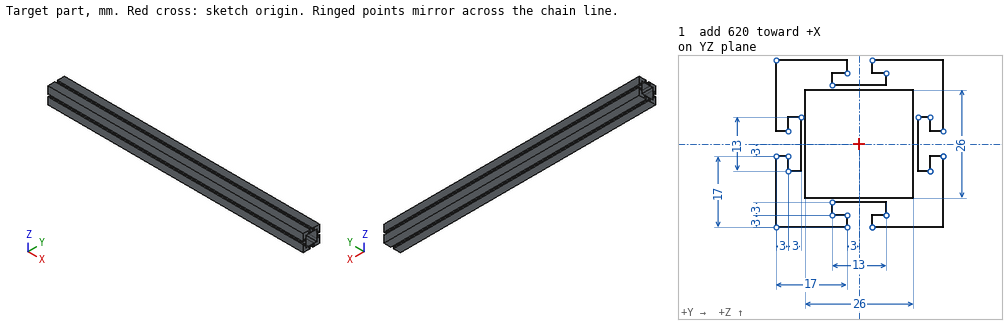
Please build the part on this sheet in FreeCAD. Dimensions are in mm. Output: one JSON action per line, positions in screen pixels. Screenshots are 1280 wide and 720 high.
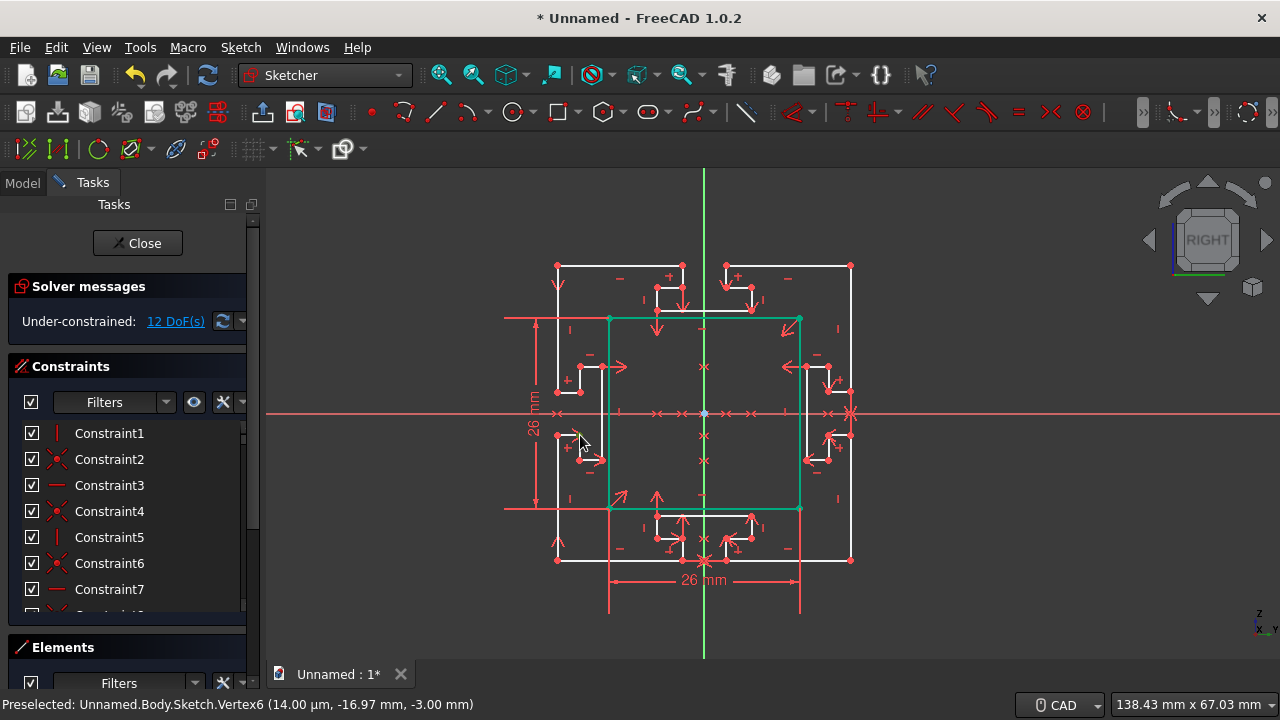
{"action": "left_click", "coordinate": [580, 393]}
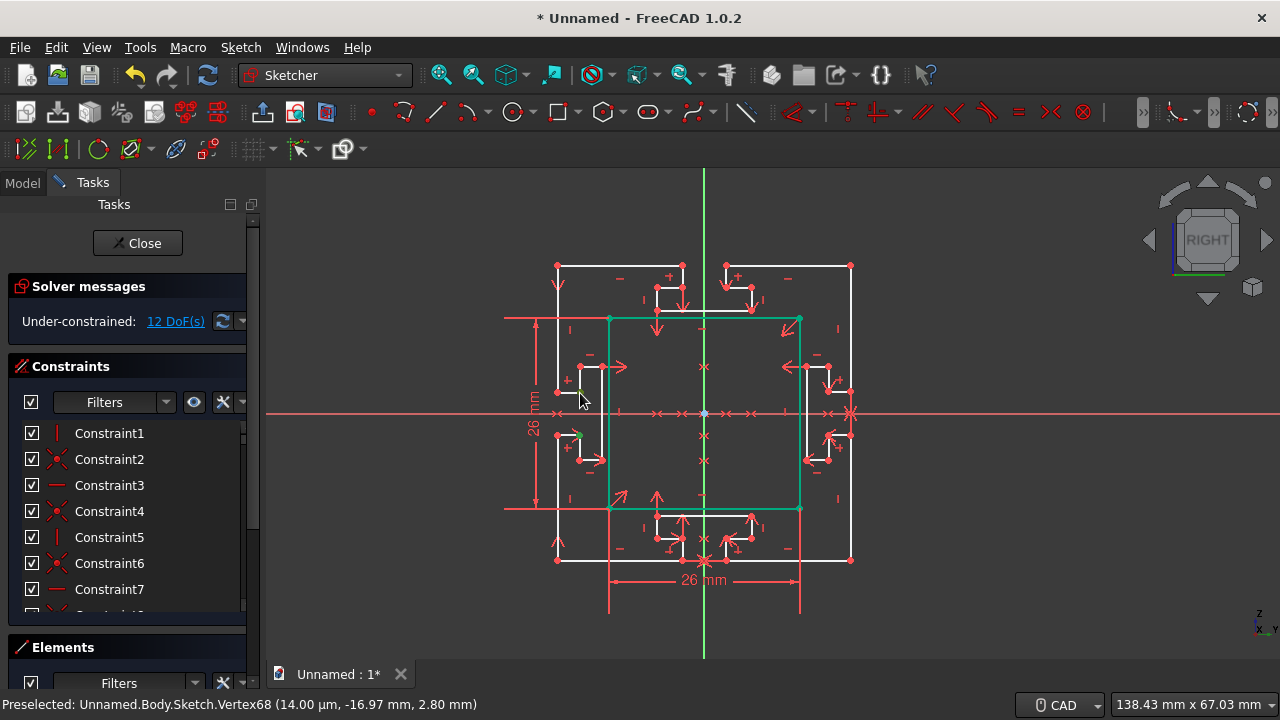
{"action": "left_click", "coordinate": [353, 414]}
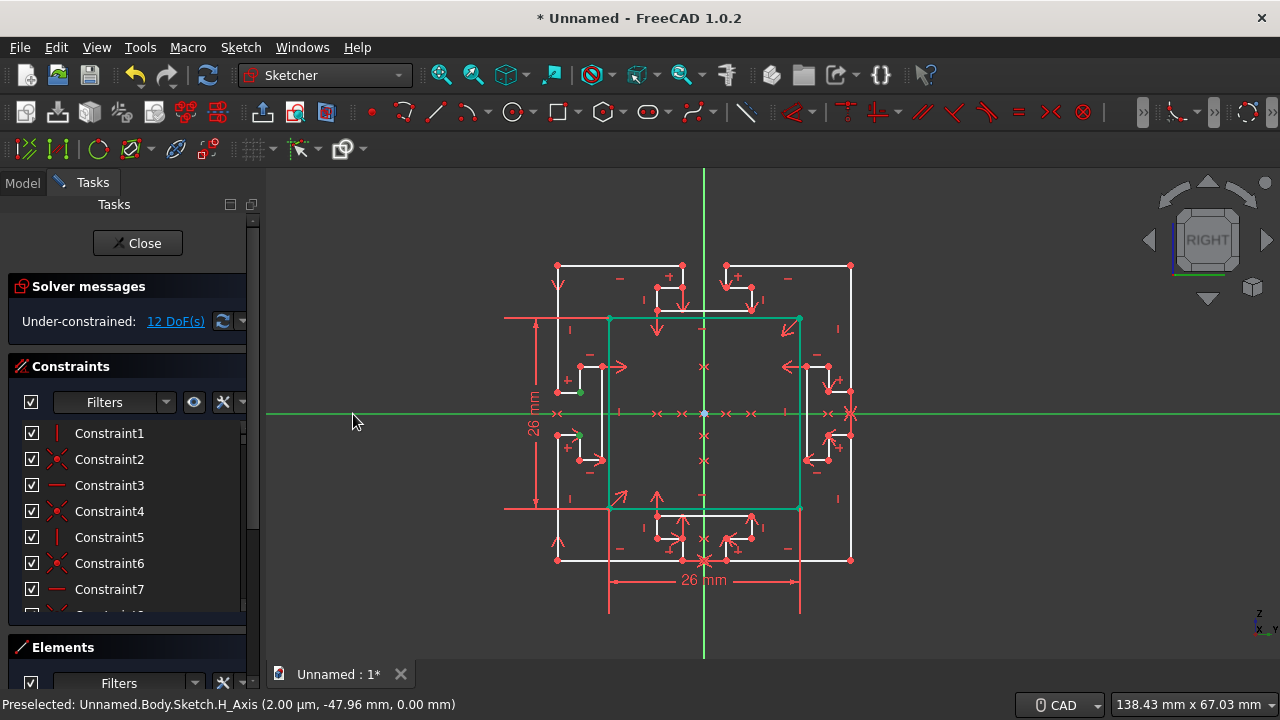
{"action": "left_click", "coordinate": [1052, 112]}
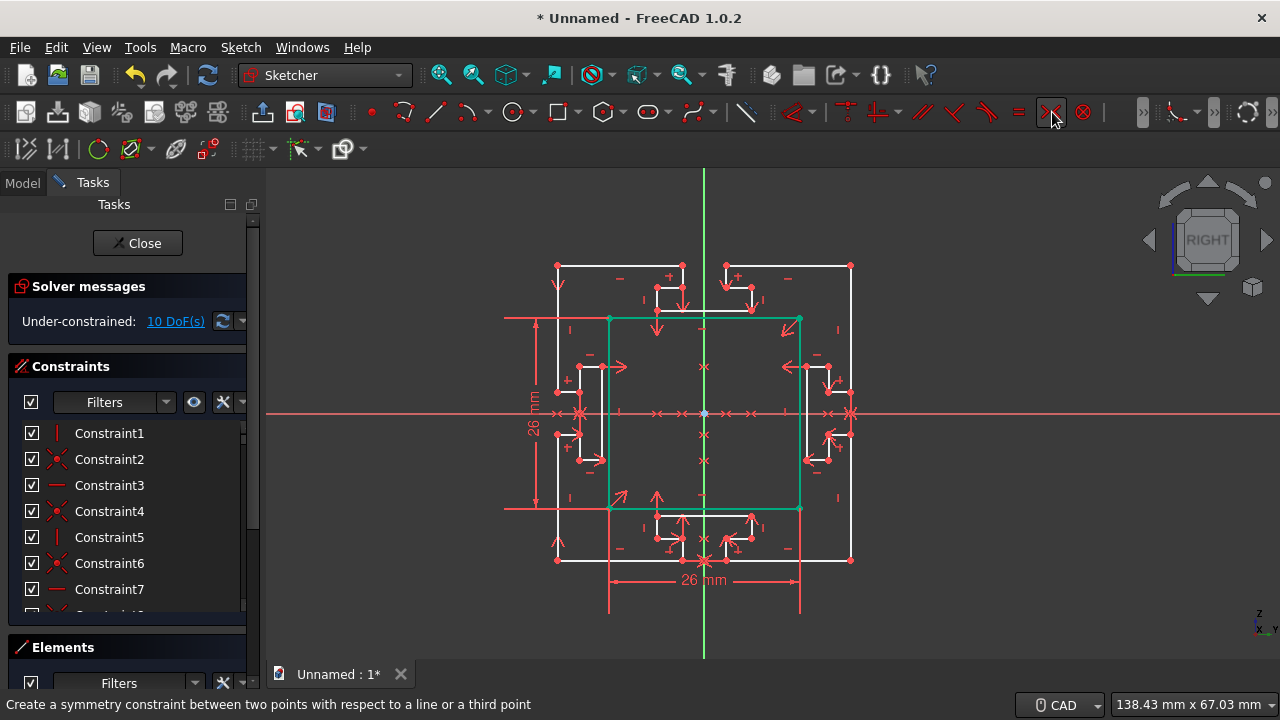
{"action": "key", "text": "d"}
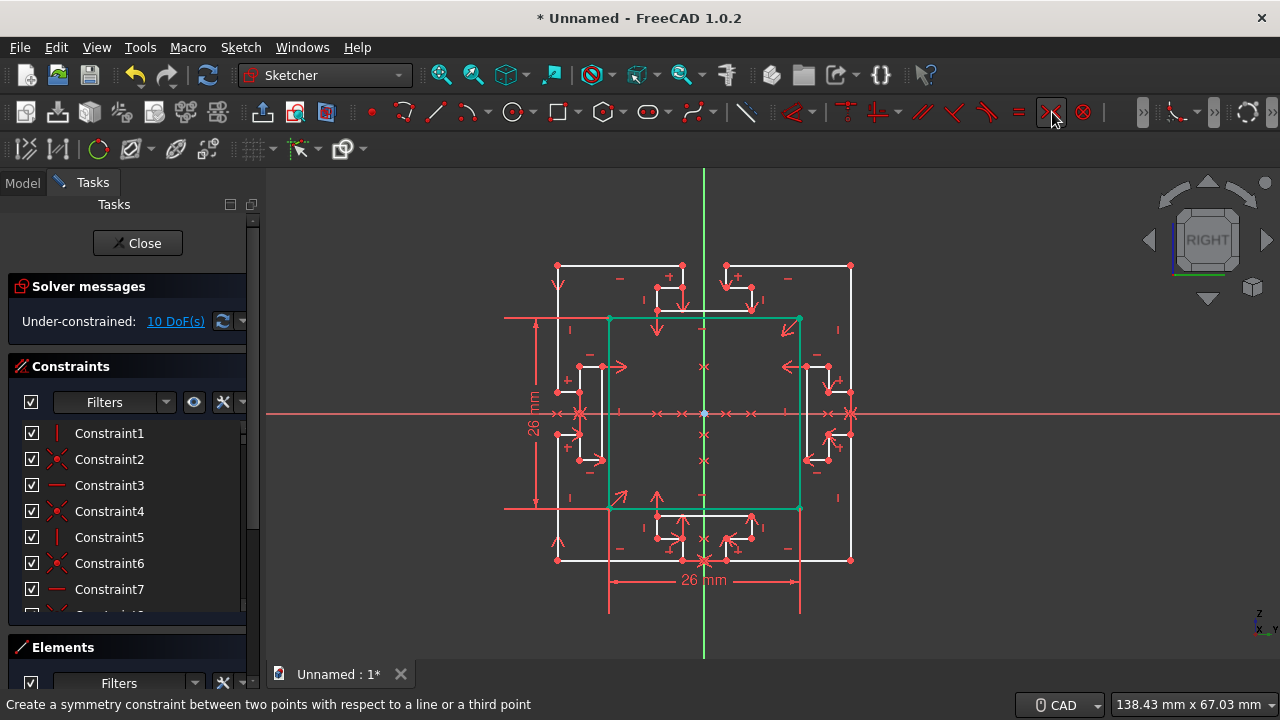
{"action": "scroll", "coordinate": [591, 460], "scroll_direction": "up", "scroll_amount": 3}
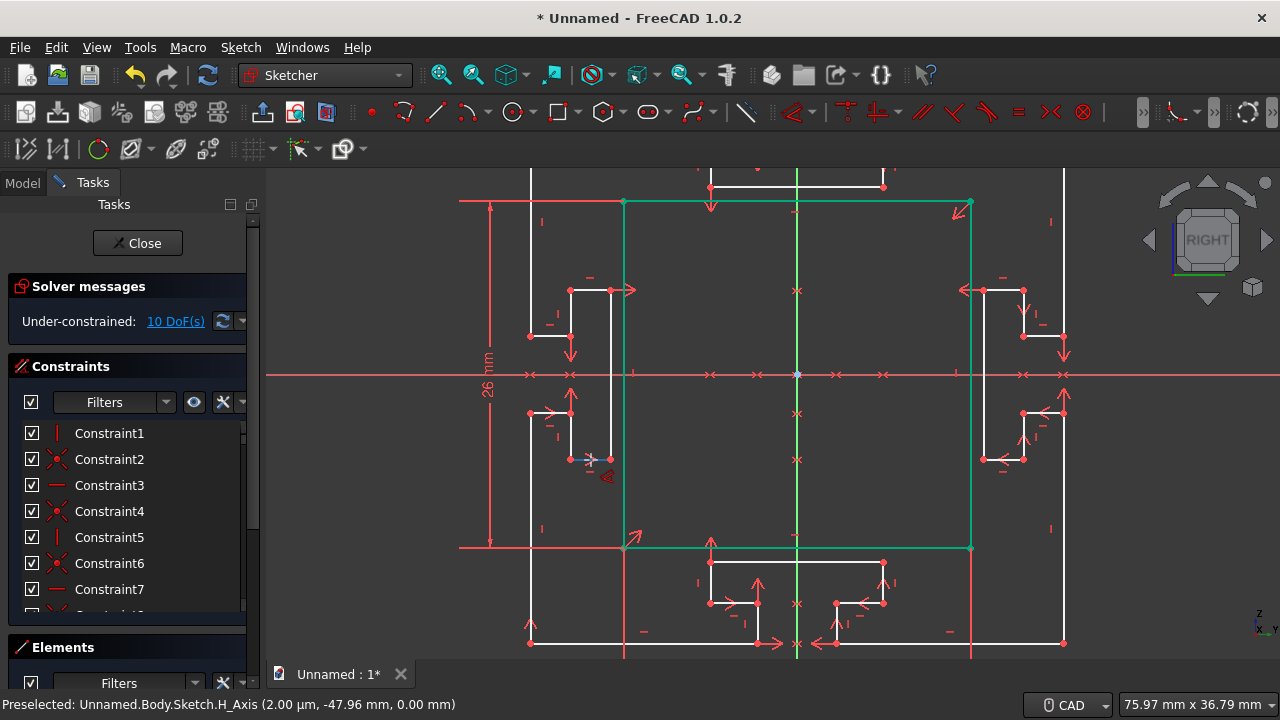
{"action": "left_click", "coordinate": [591, 460]}
{"action": "left_click", "coordinate": [591, 494]}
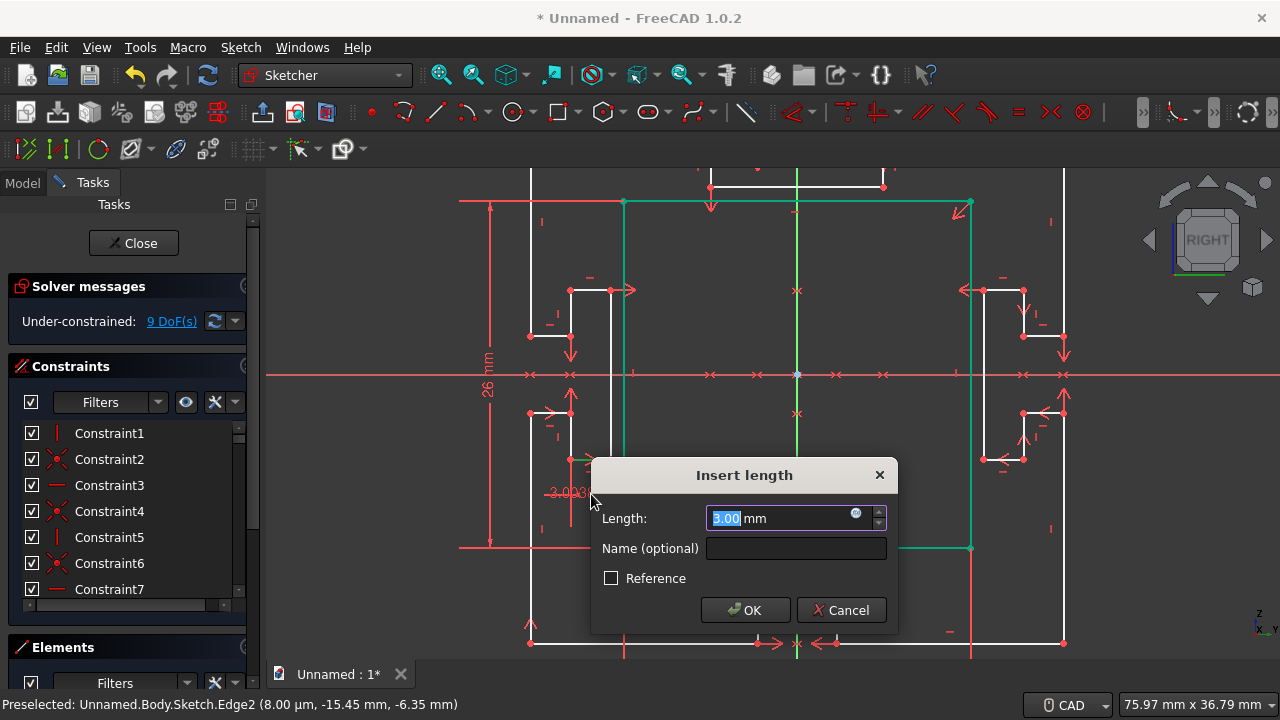
{"action": "type", "text": "3"}
{"action": "key", "text": "Return"}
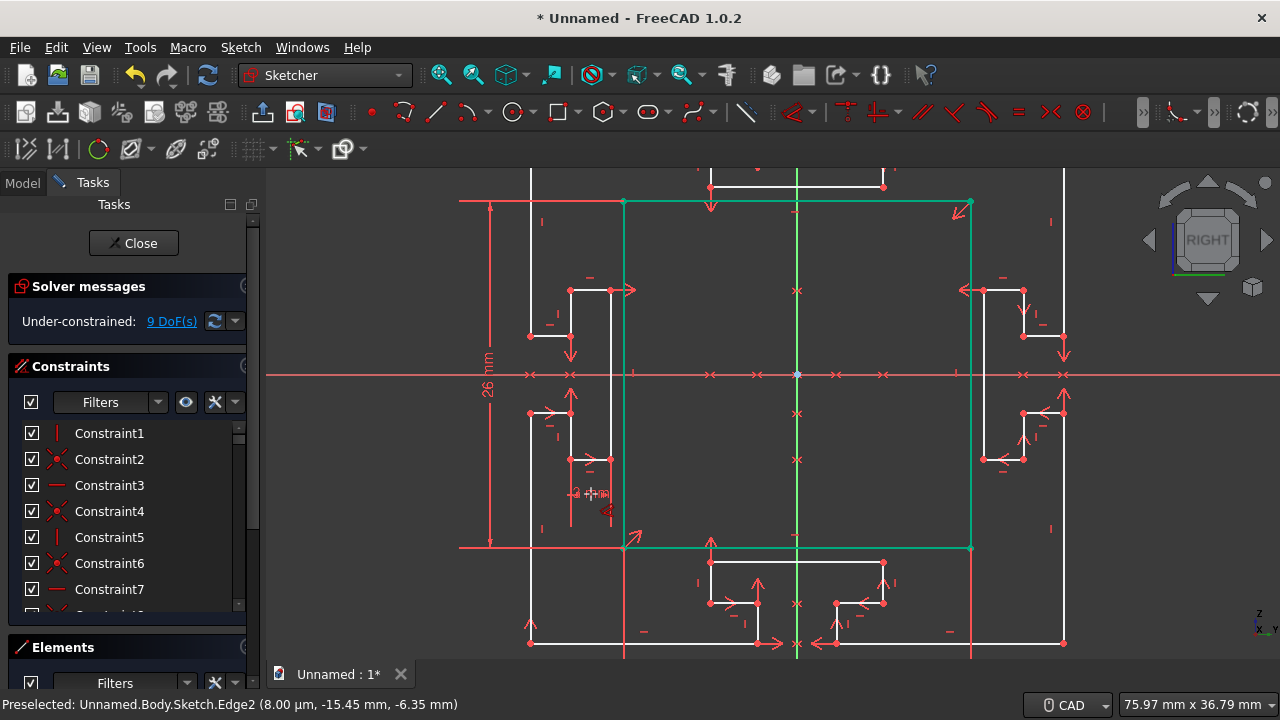
{"action": "left_click", "coordinate": [559, 413]}
{"action": "left_click", "coordinate": [551, 447]}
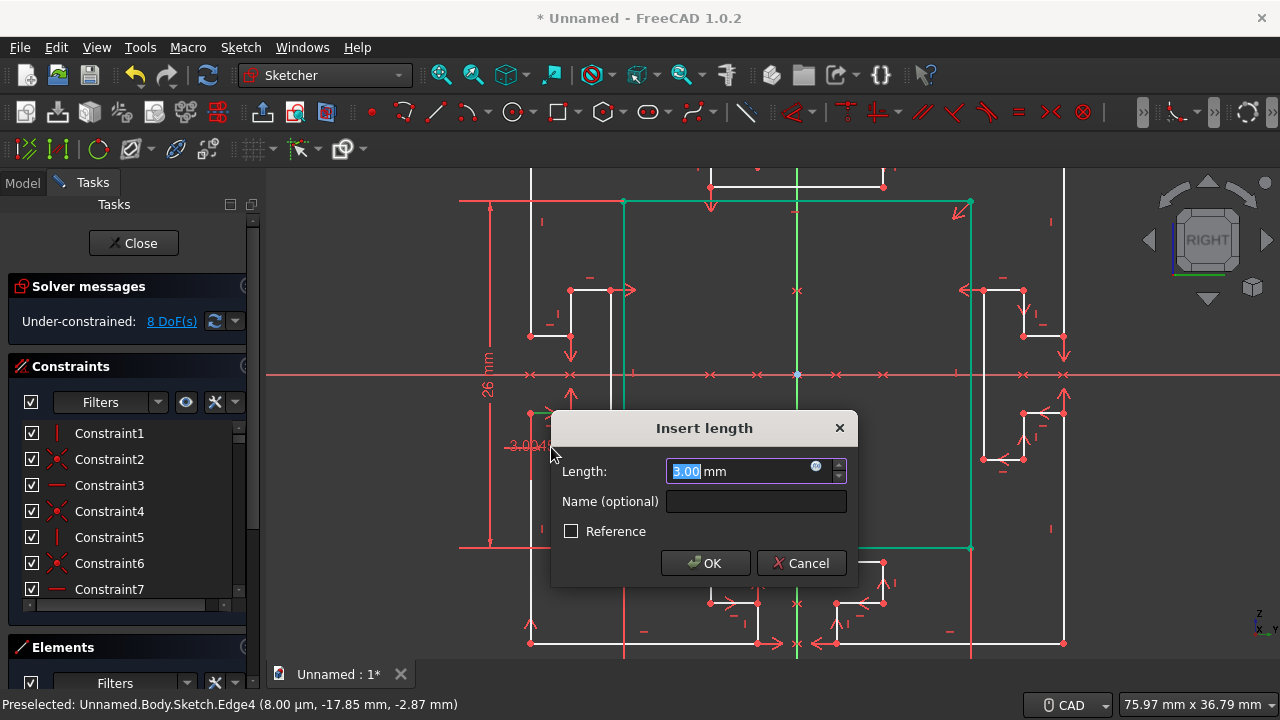
{"action": "type", "text": "3"}
{"action": "key", "text": "Return"}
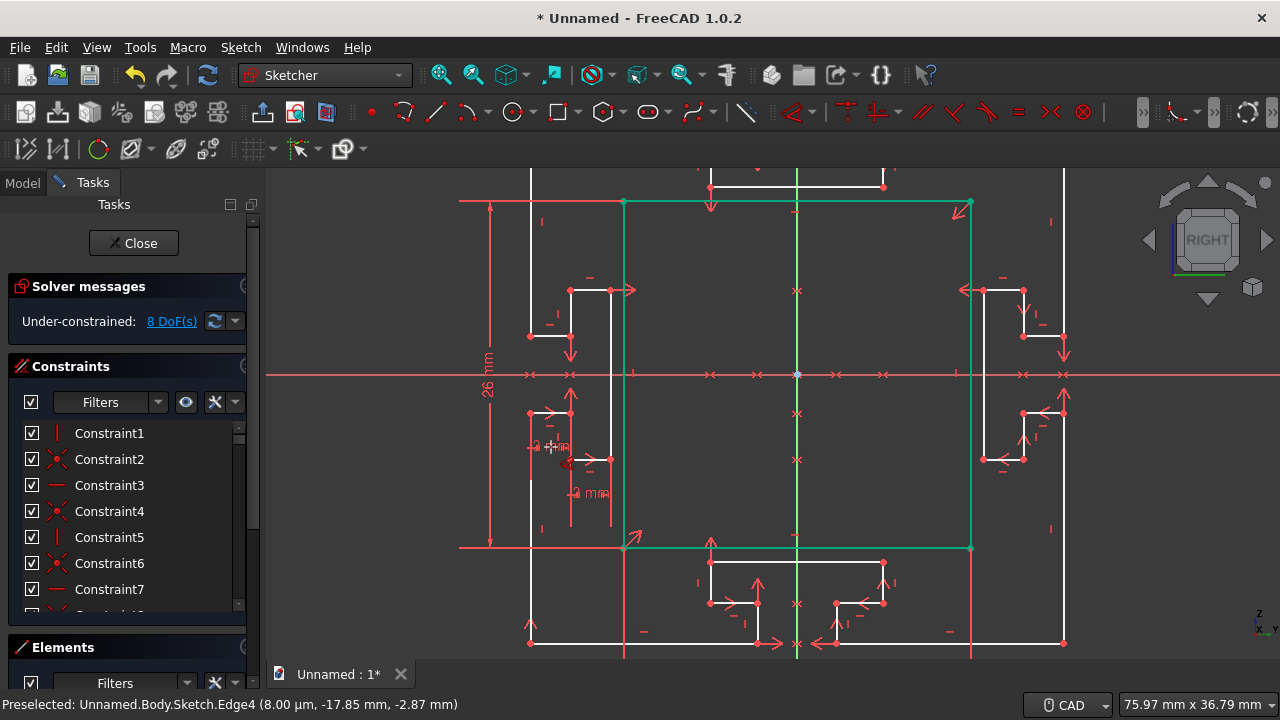
{"action": "left_click", "coordinate": [758, 615]}
{"action": "left_click", "coordinate": [724, 617]}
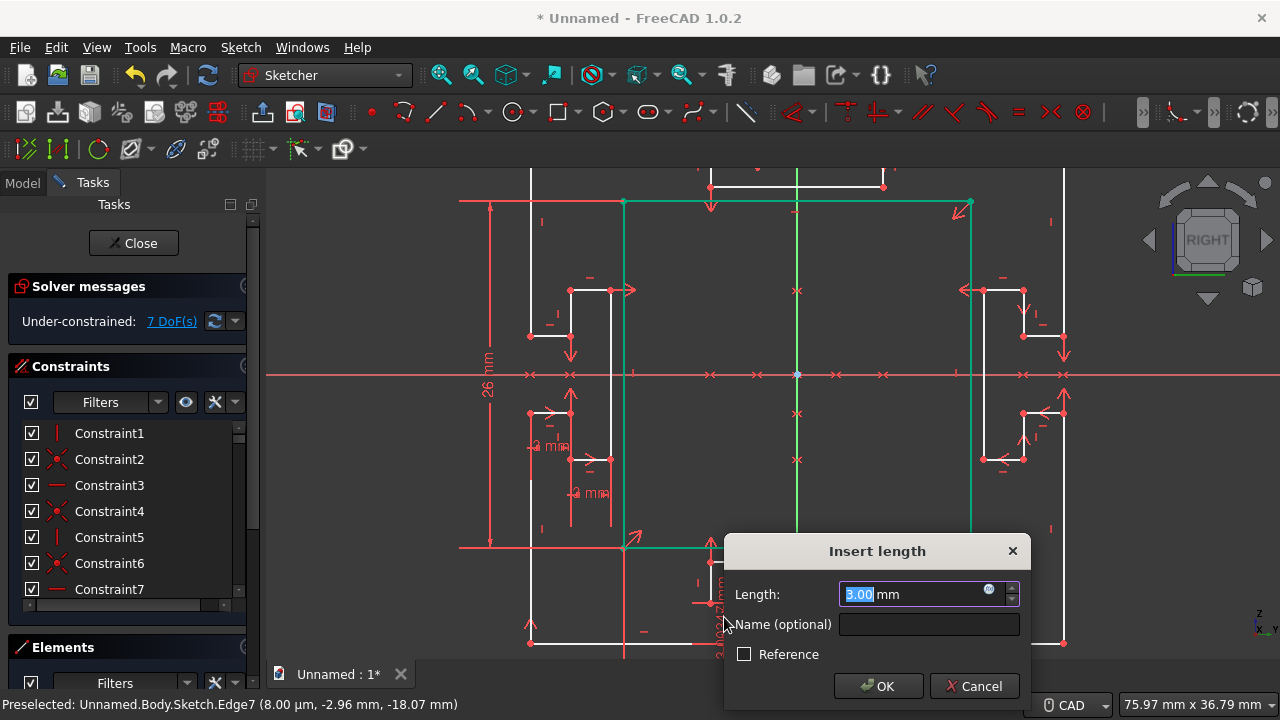
{"action": "type", "text": "3"}
{"action": "key", "text": "Return"}